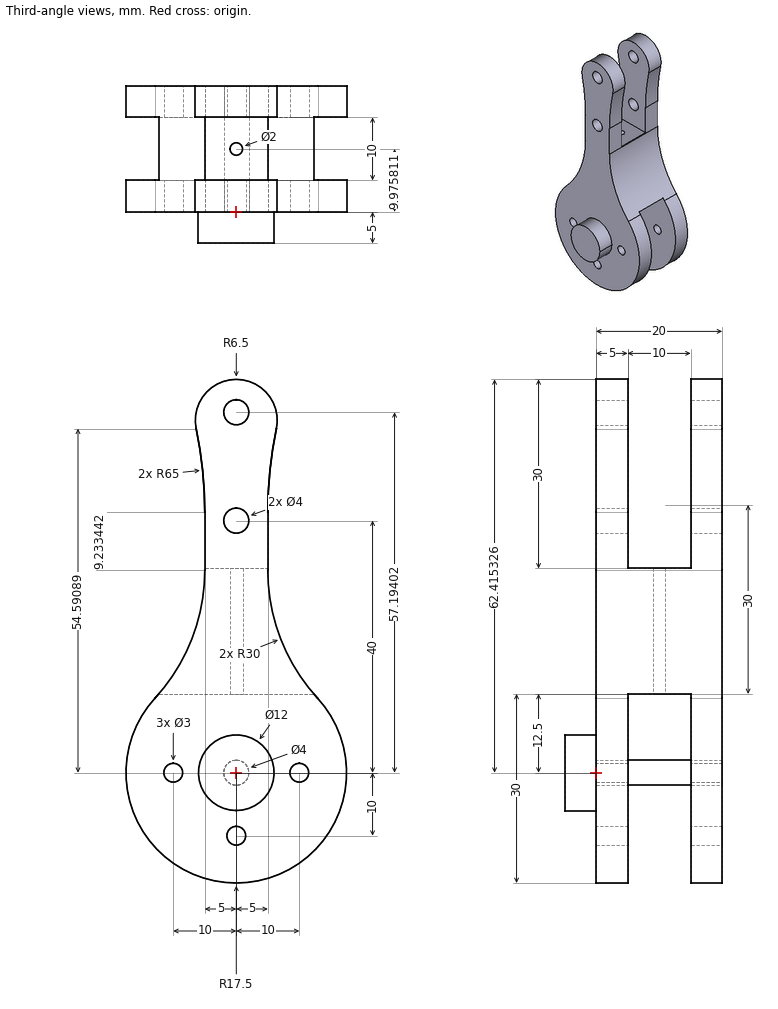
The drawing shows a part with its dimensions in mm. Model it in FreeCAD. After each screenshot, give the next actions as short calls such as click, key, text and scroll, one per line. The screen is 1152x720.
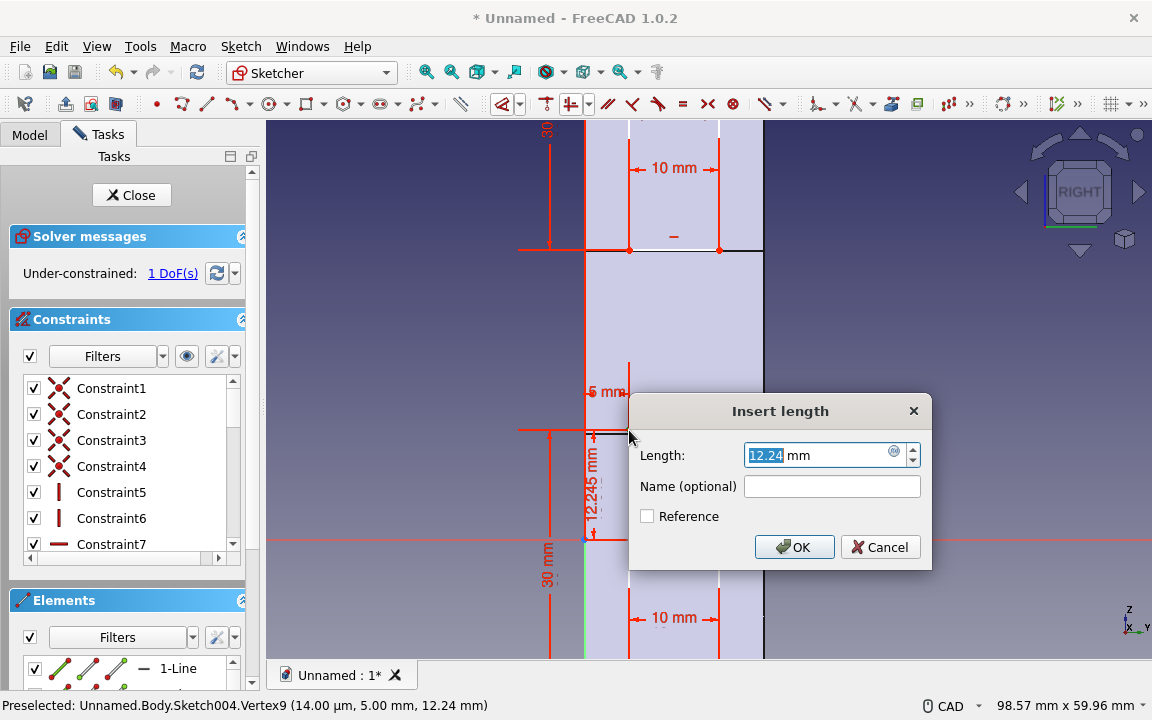
text(12.5)
key(Return)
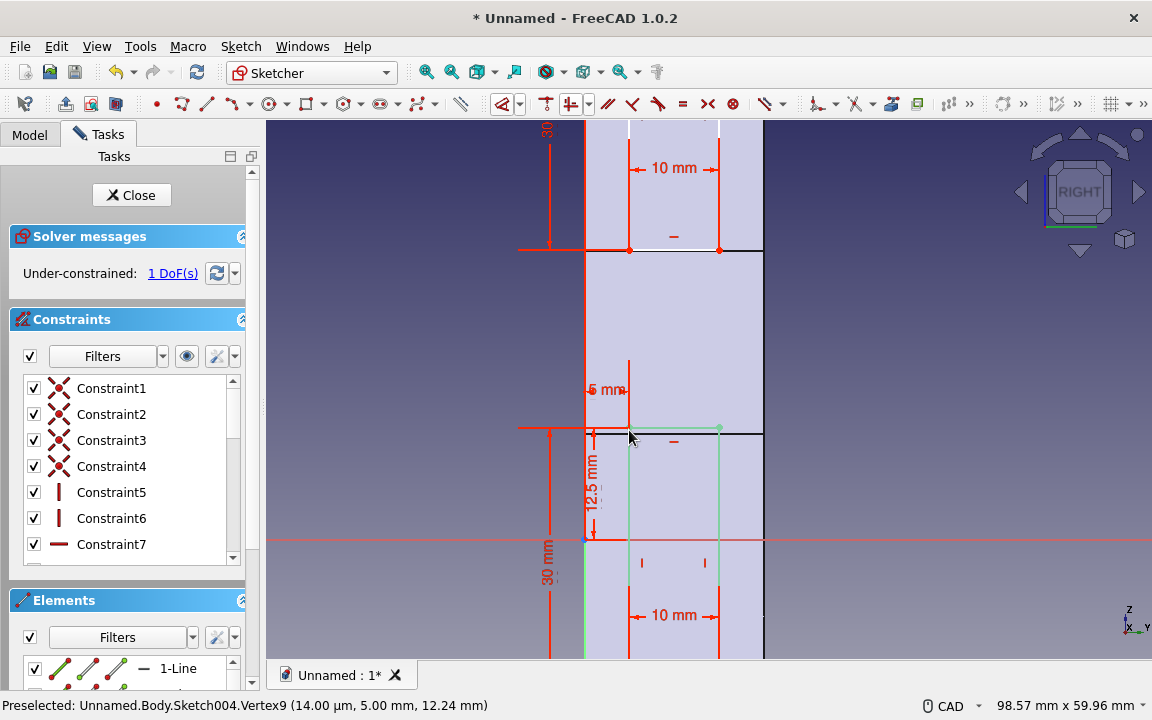
scroll(631, 431, down, 4)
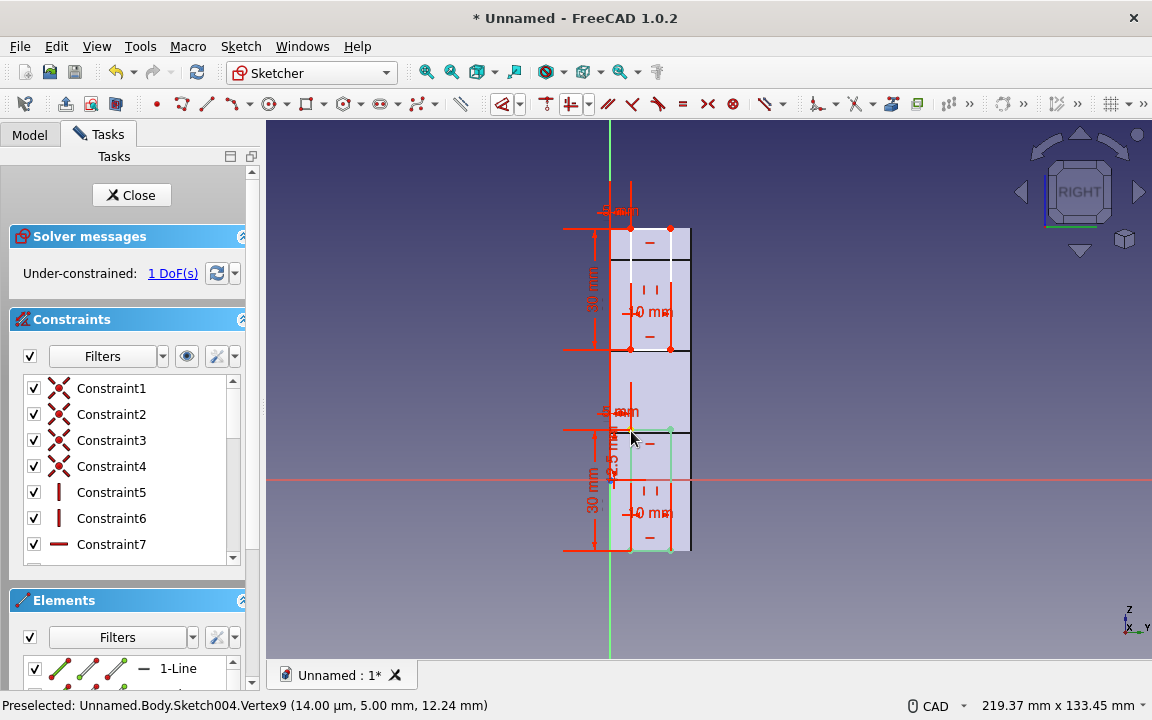
click(631, 229)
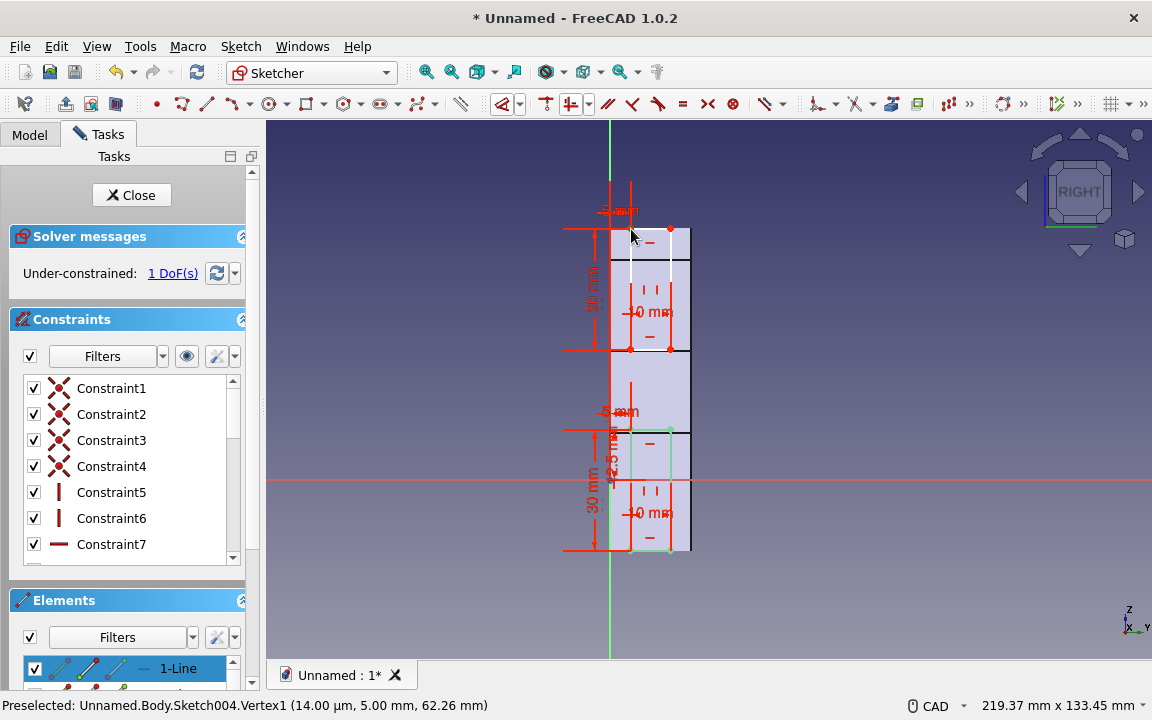
key(i)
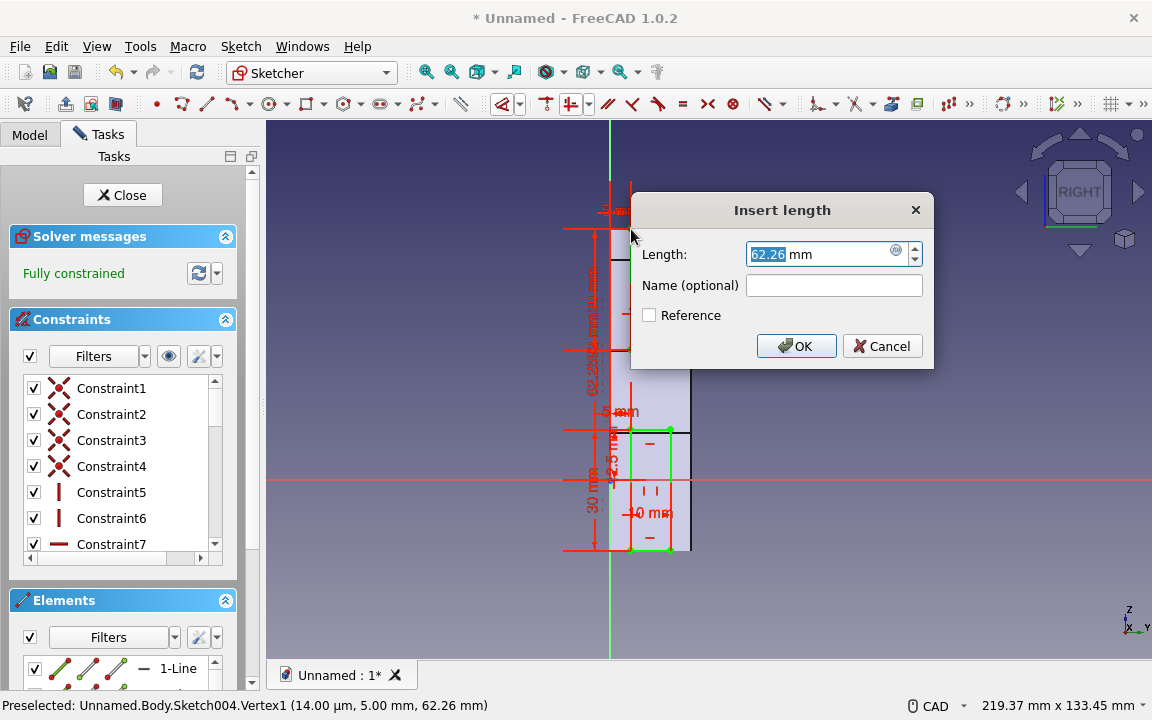
text(62.415326)
key(Return)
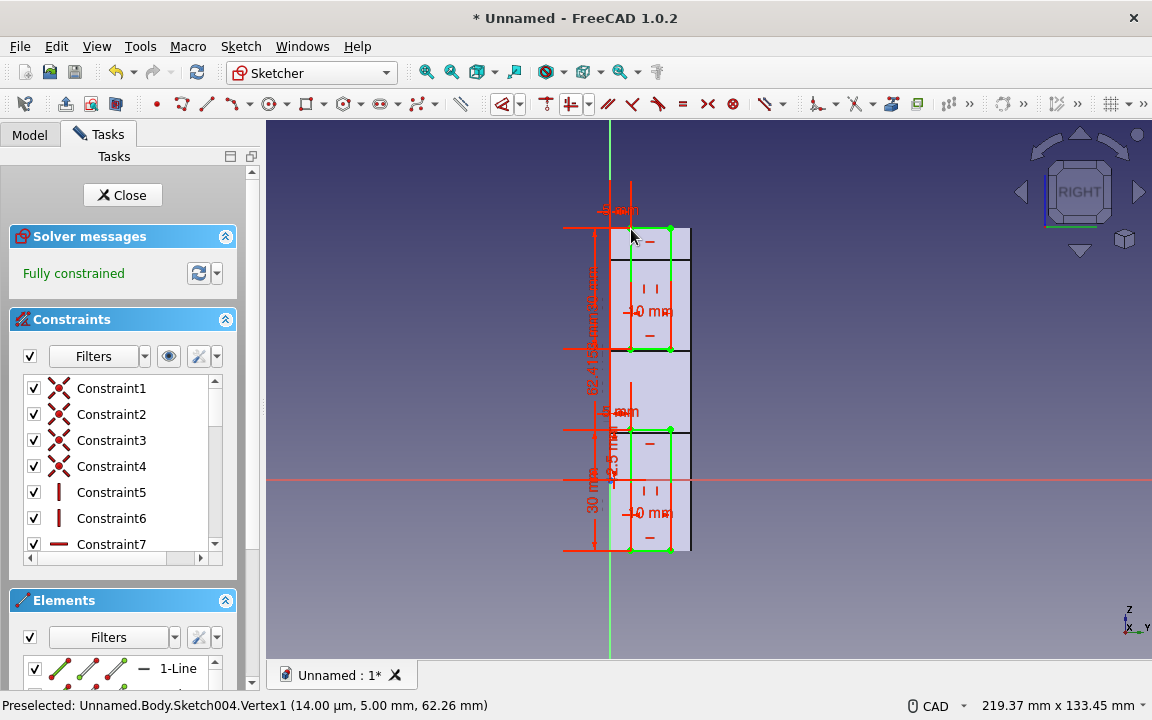
click(123, 195)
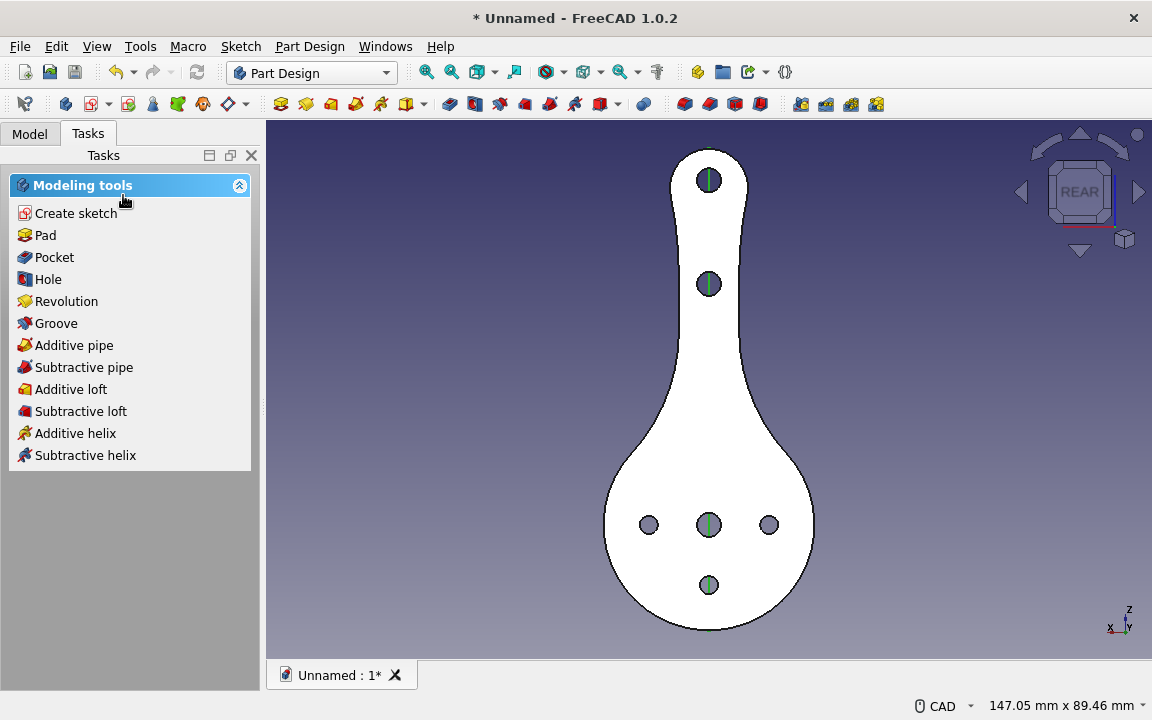
click(450, 104)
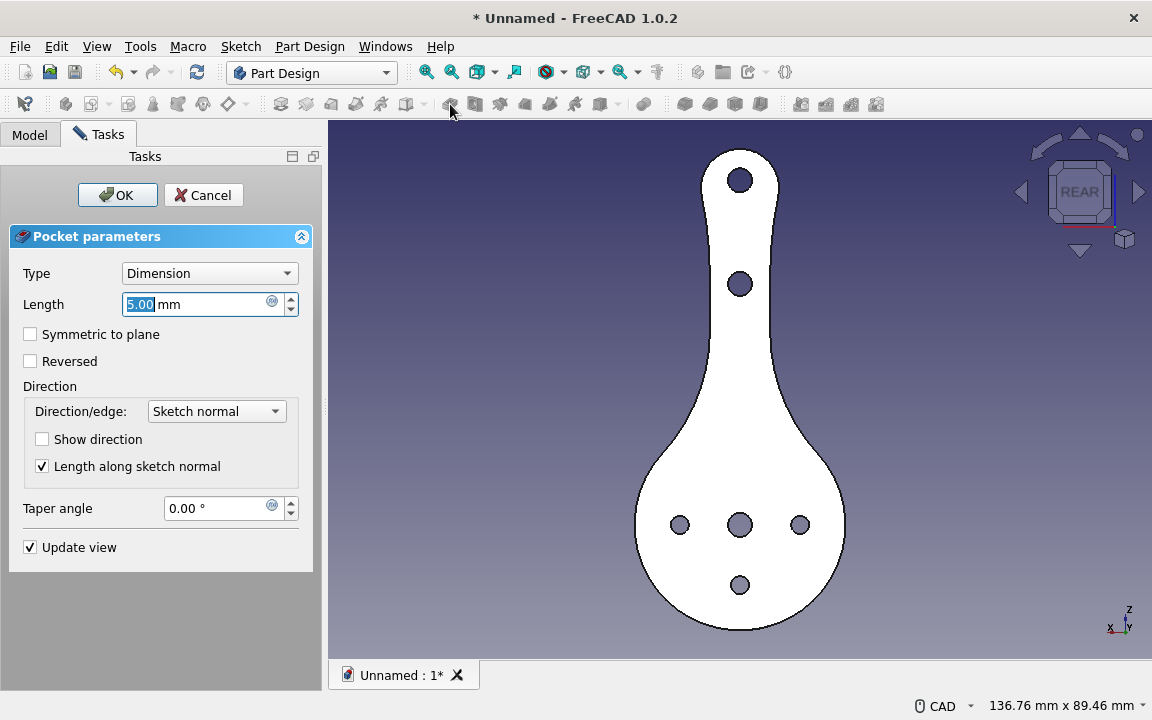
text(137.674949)
key(Tab)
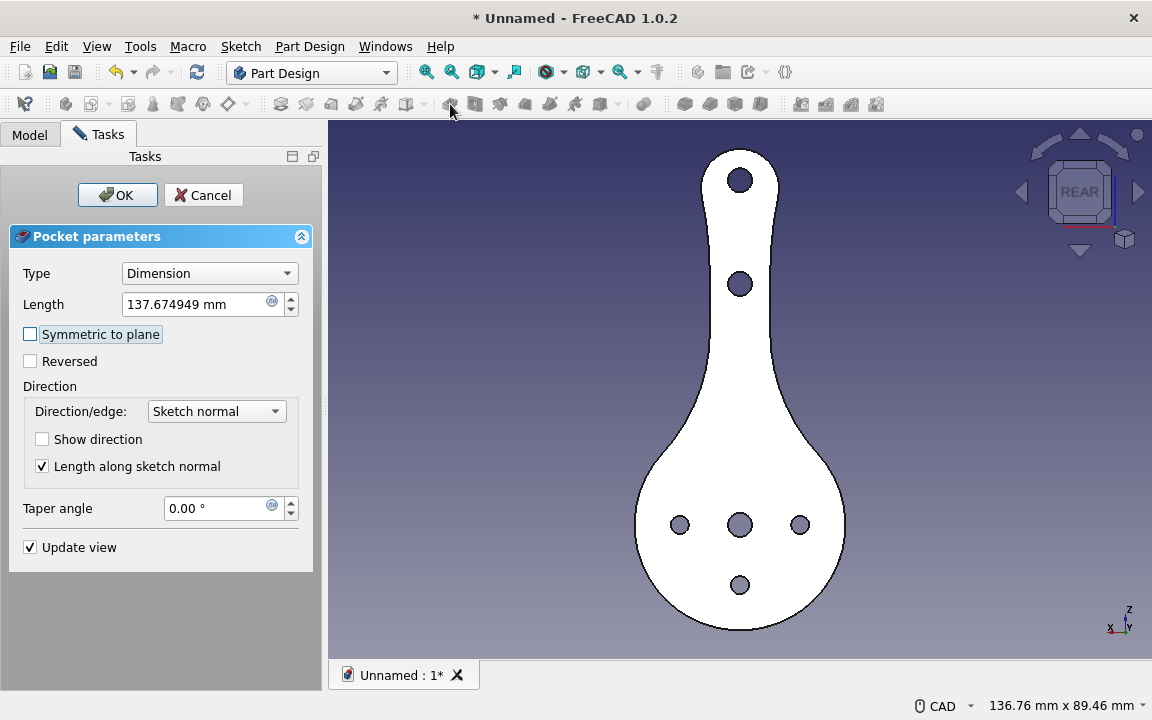
click(31, 334)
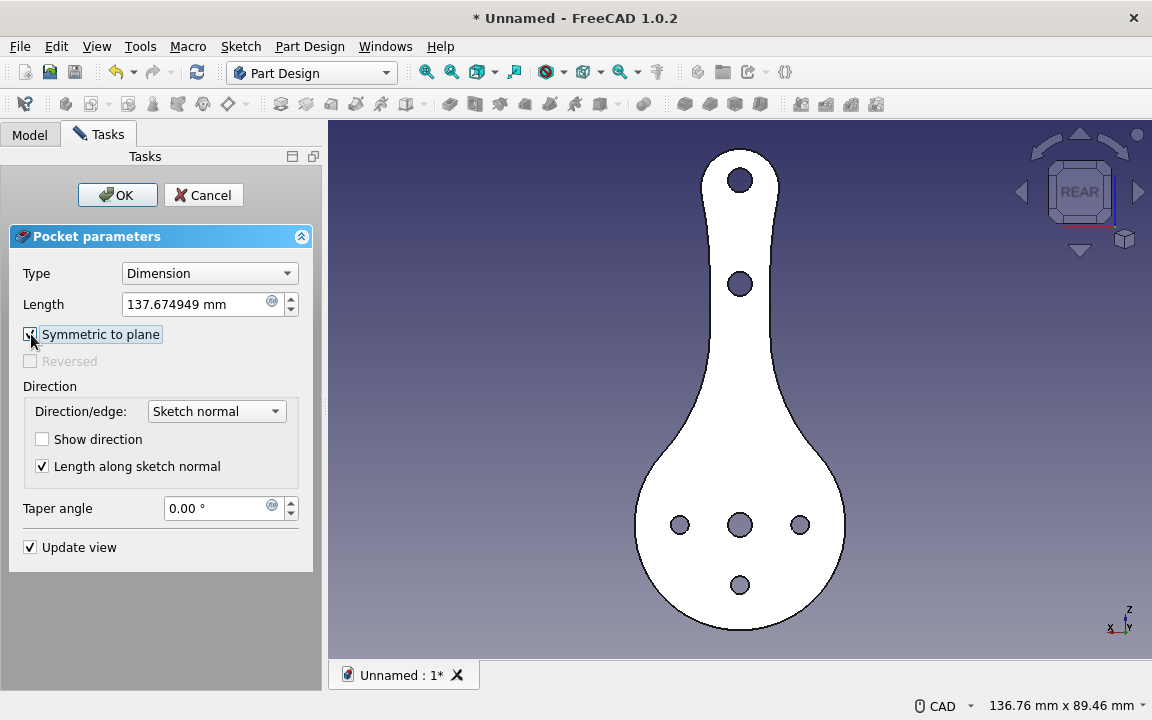
click(118, 195)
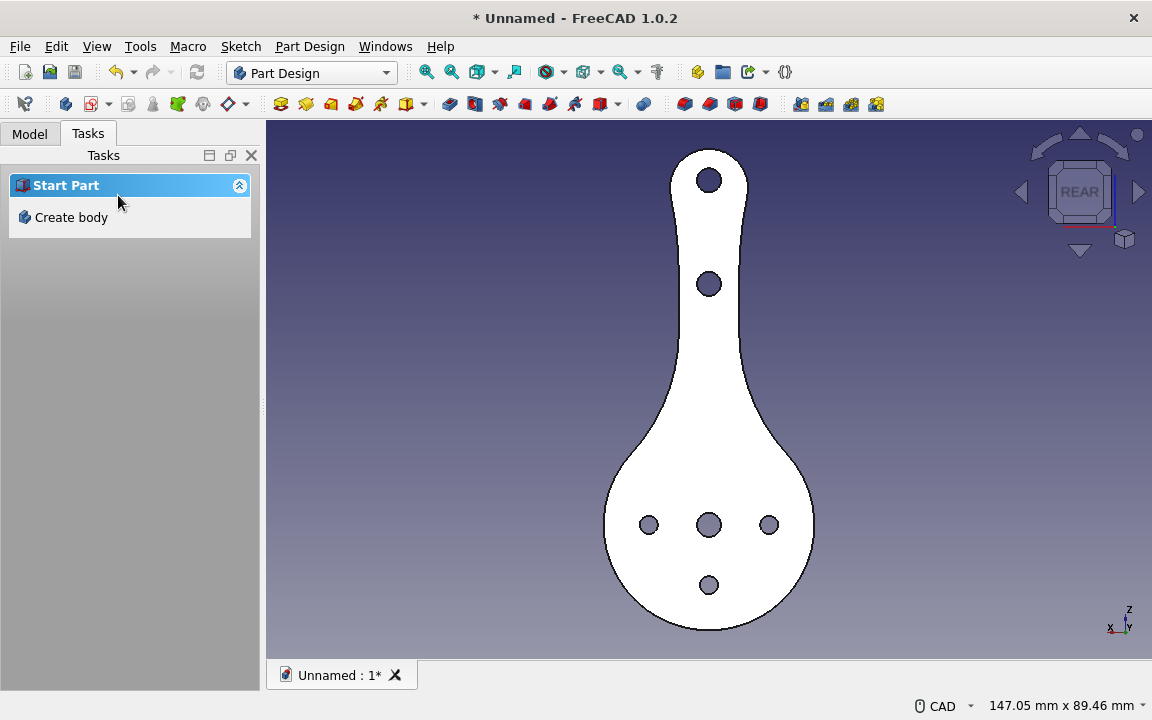
click(90, 104)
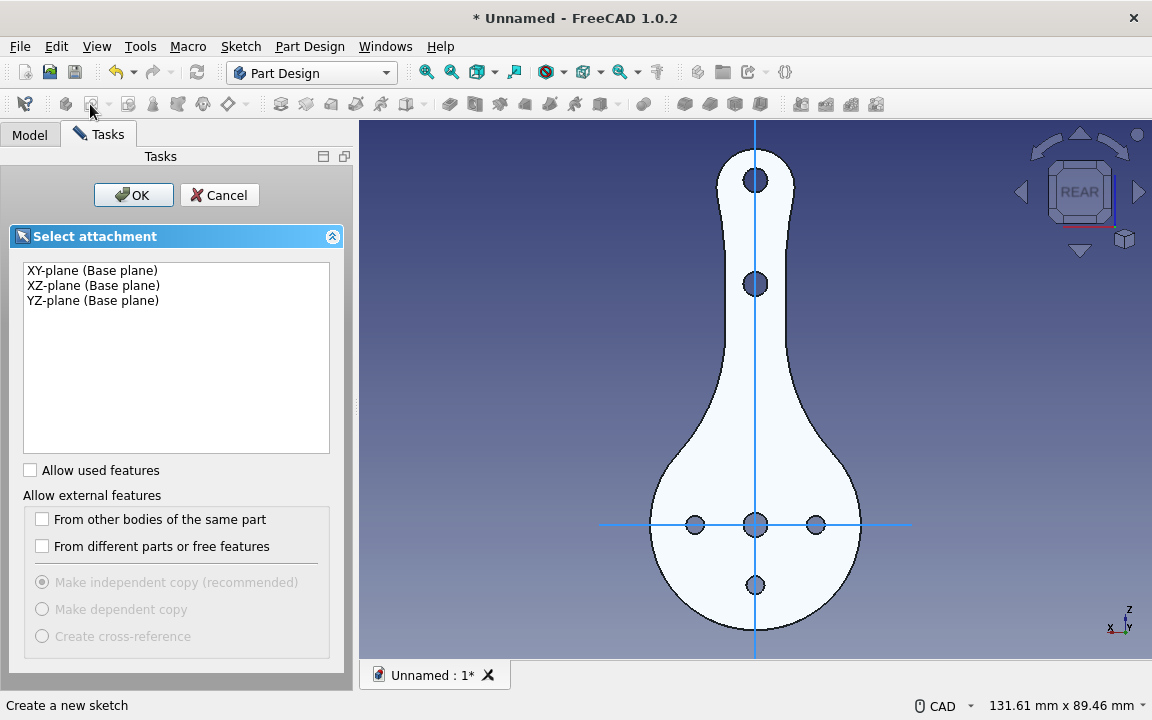
click(84, 286)